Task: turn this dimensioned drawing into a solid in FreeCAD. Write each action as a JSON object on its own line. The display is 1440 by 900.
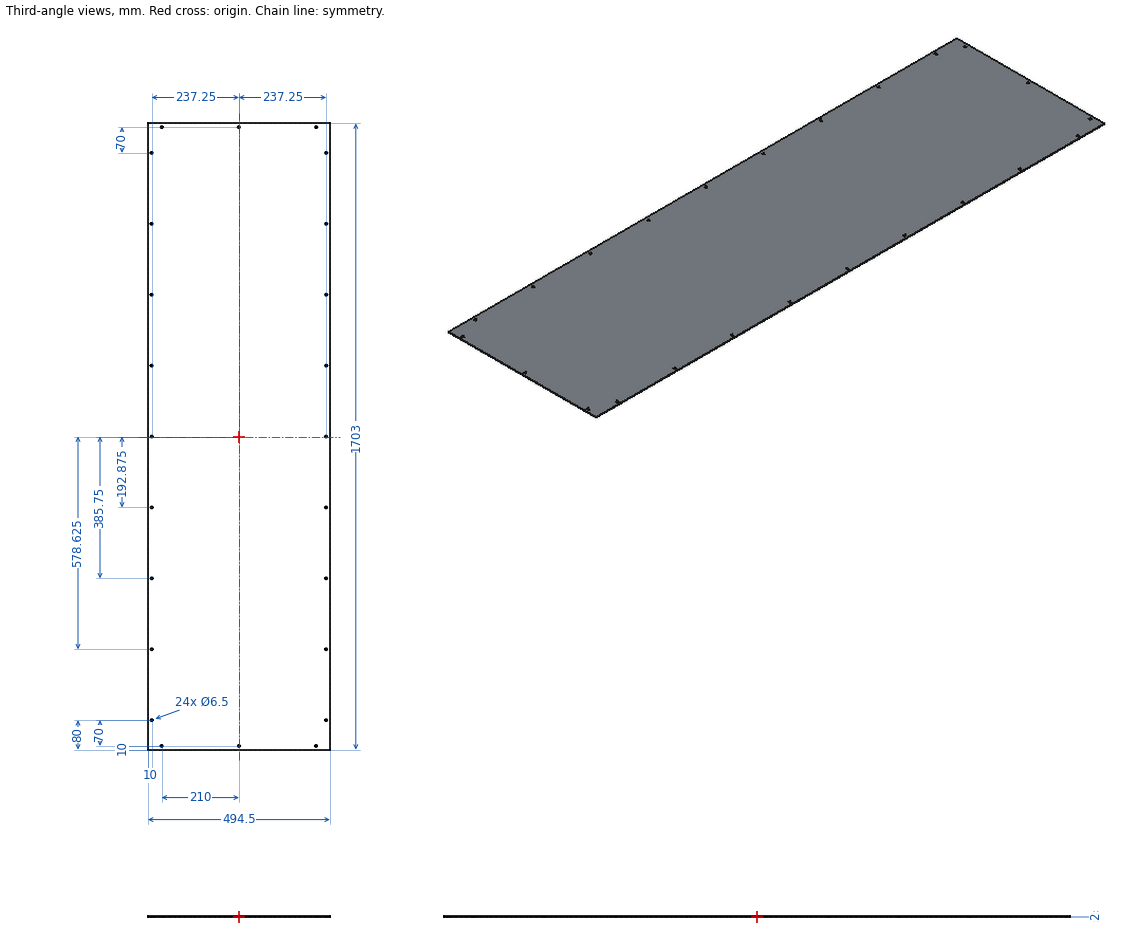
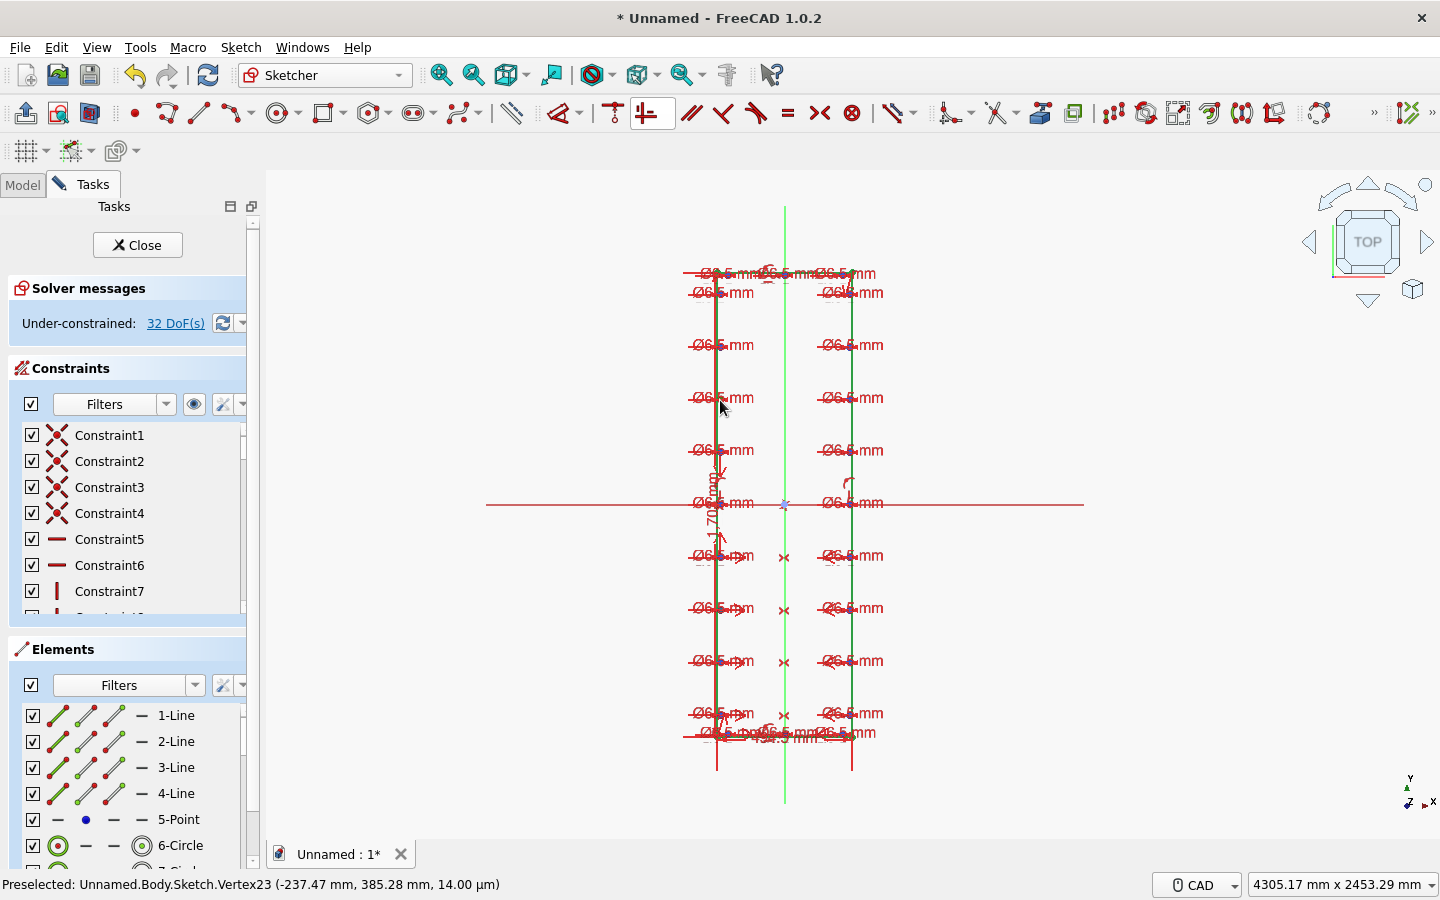
{"action": "left_click", "coordinate": [504, 505]}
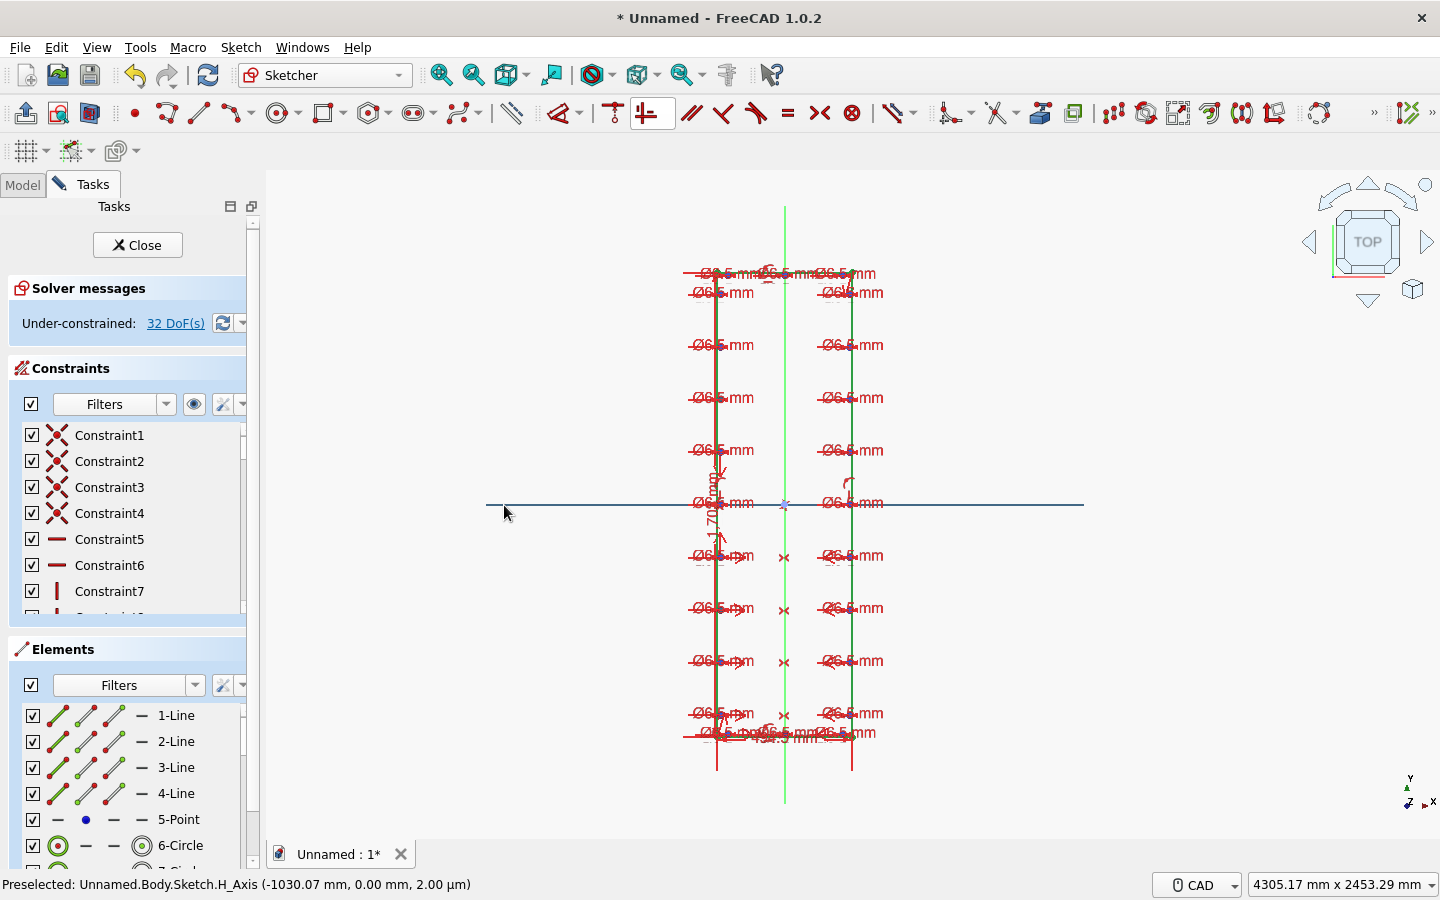
{"action": "left_click", "coordinate": [820, 114]}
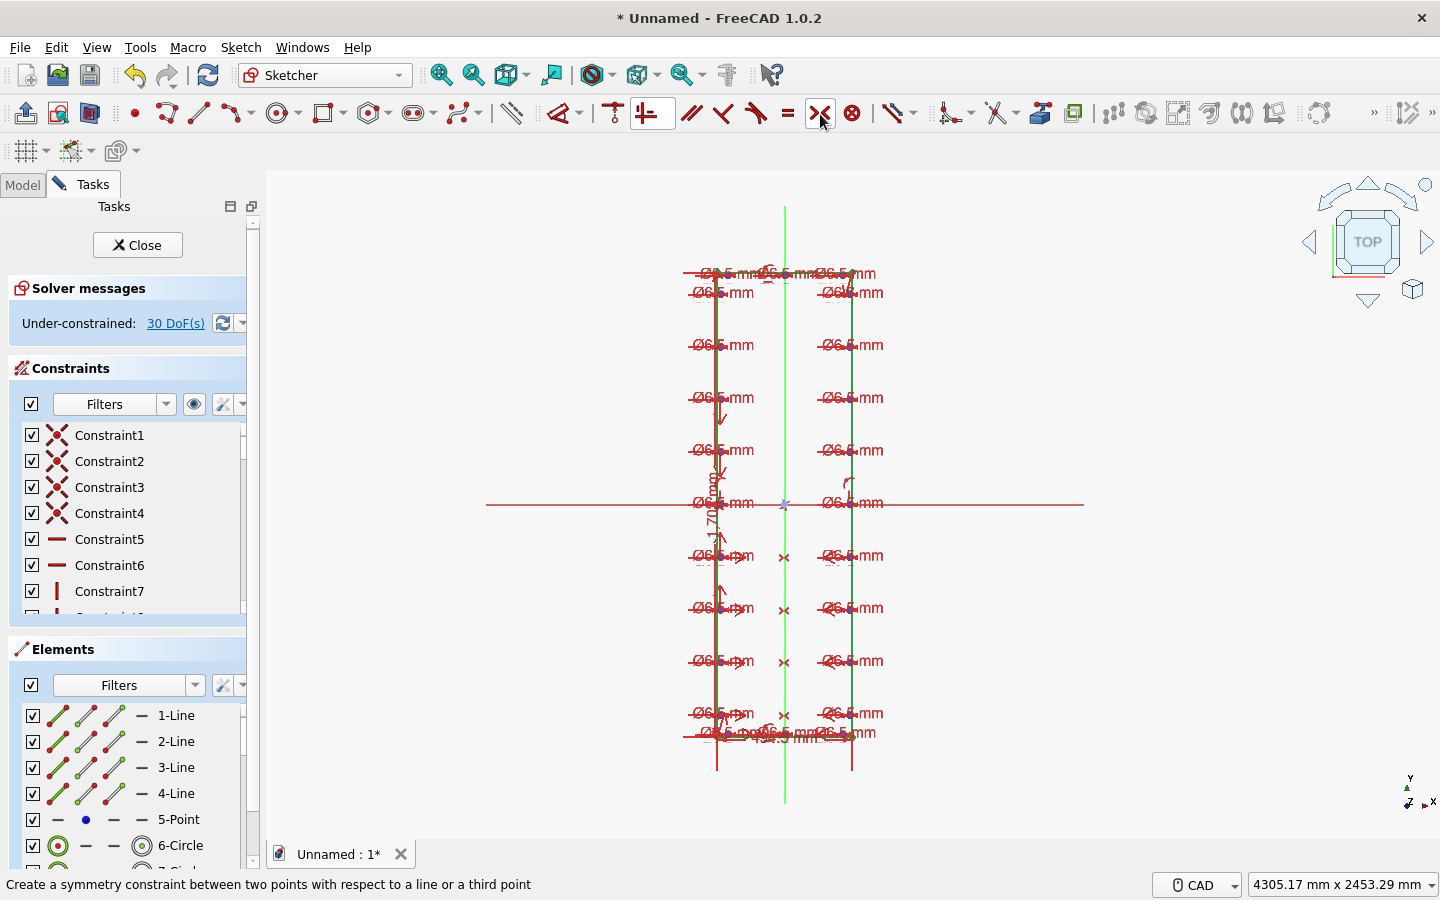
{"action": "left_click", "coordinate": [720, 663]}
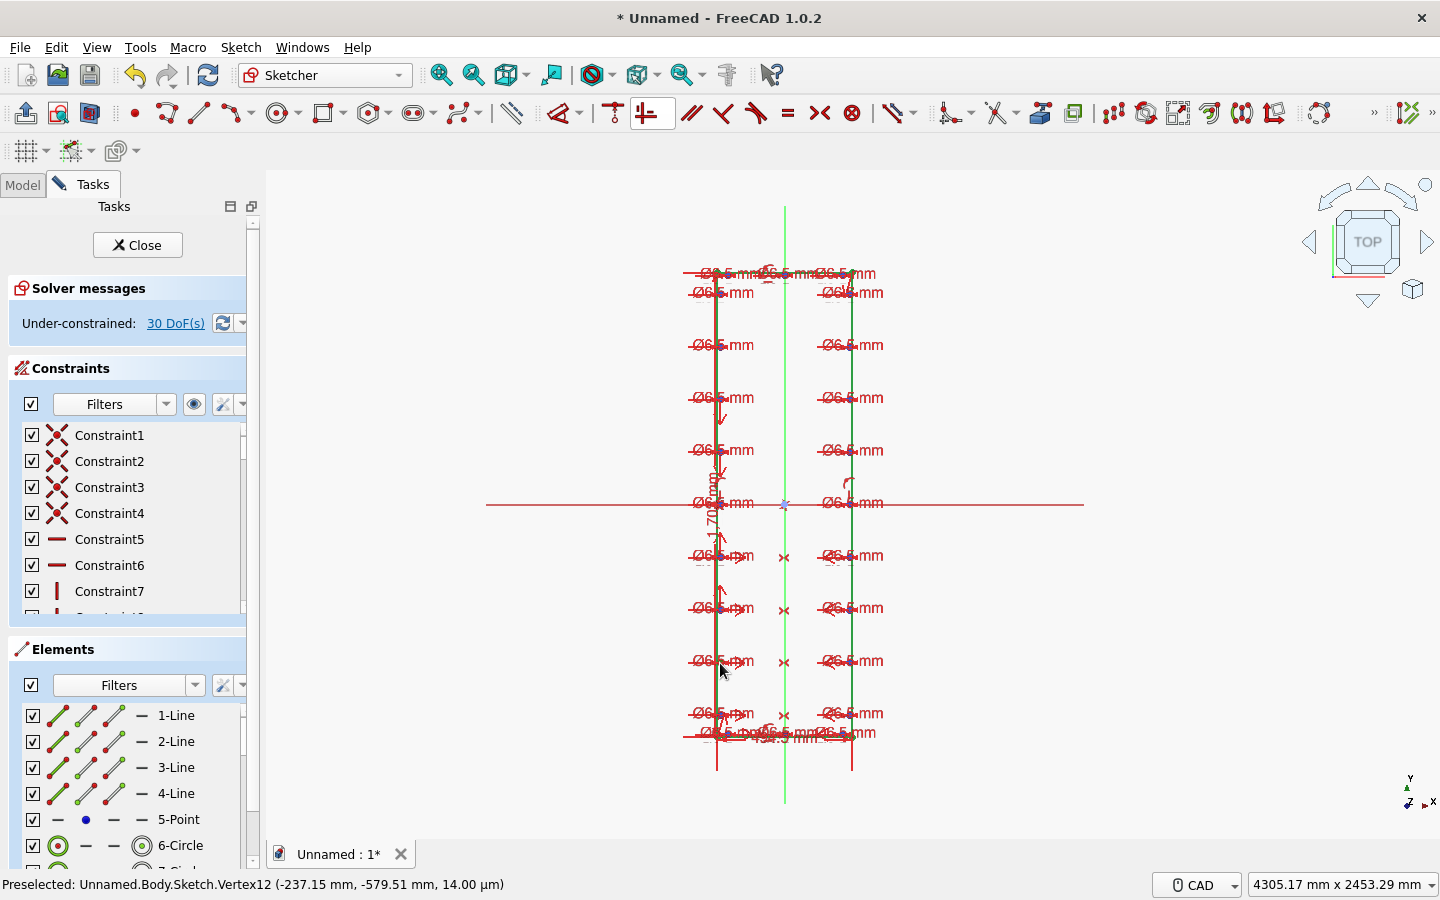
{"action": "left_click", "coordinate": [720, 347]}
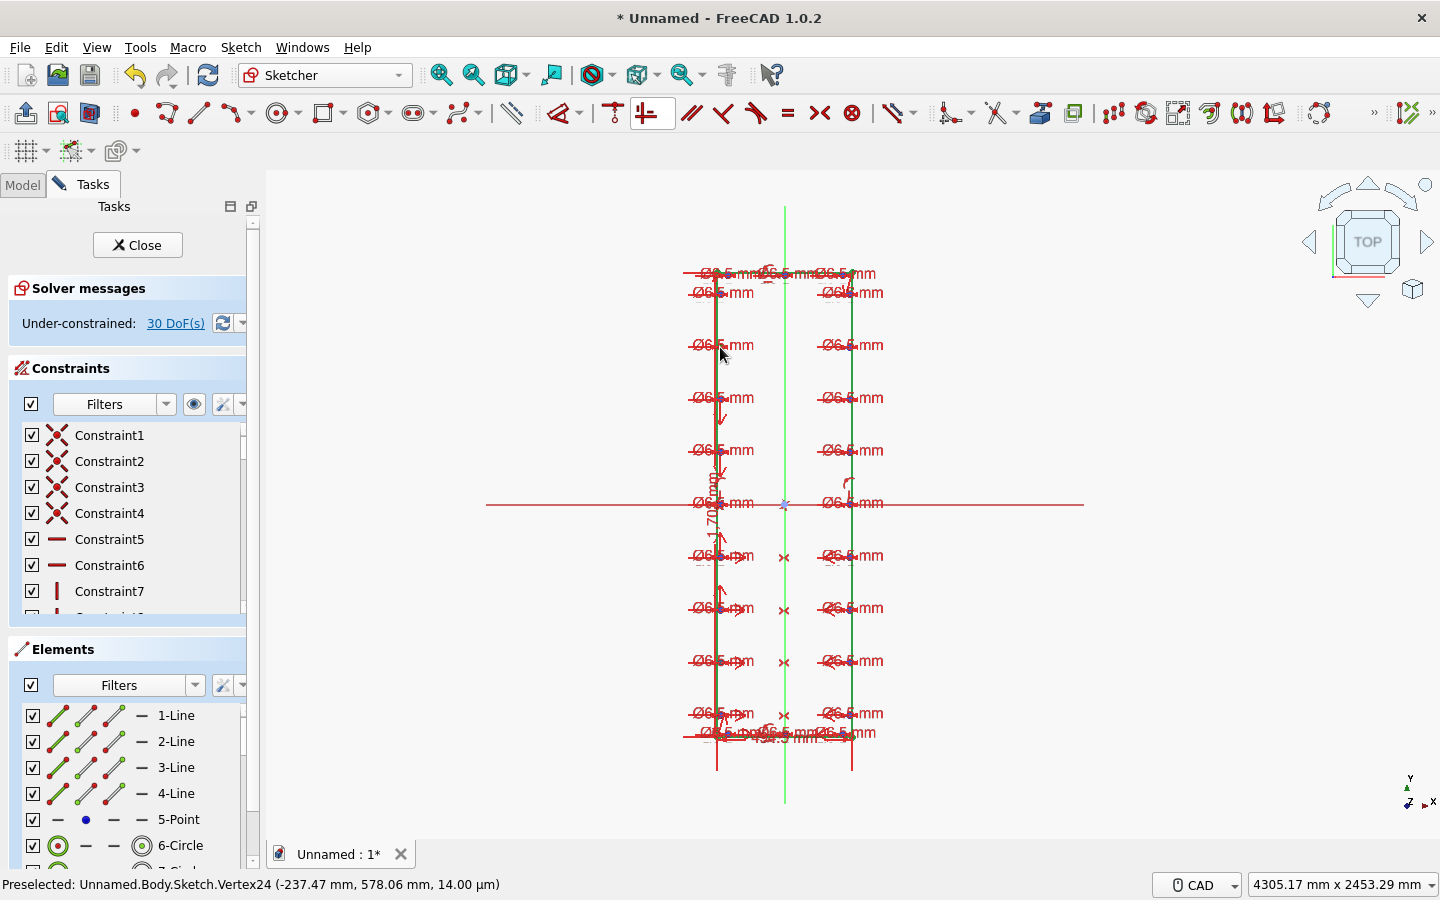
{"action": "left_click", "coordinate": [504, 505]}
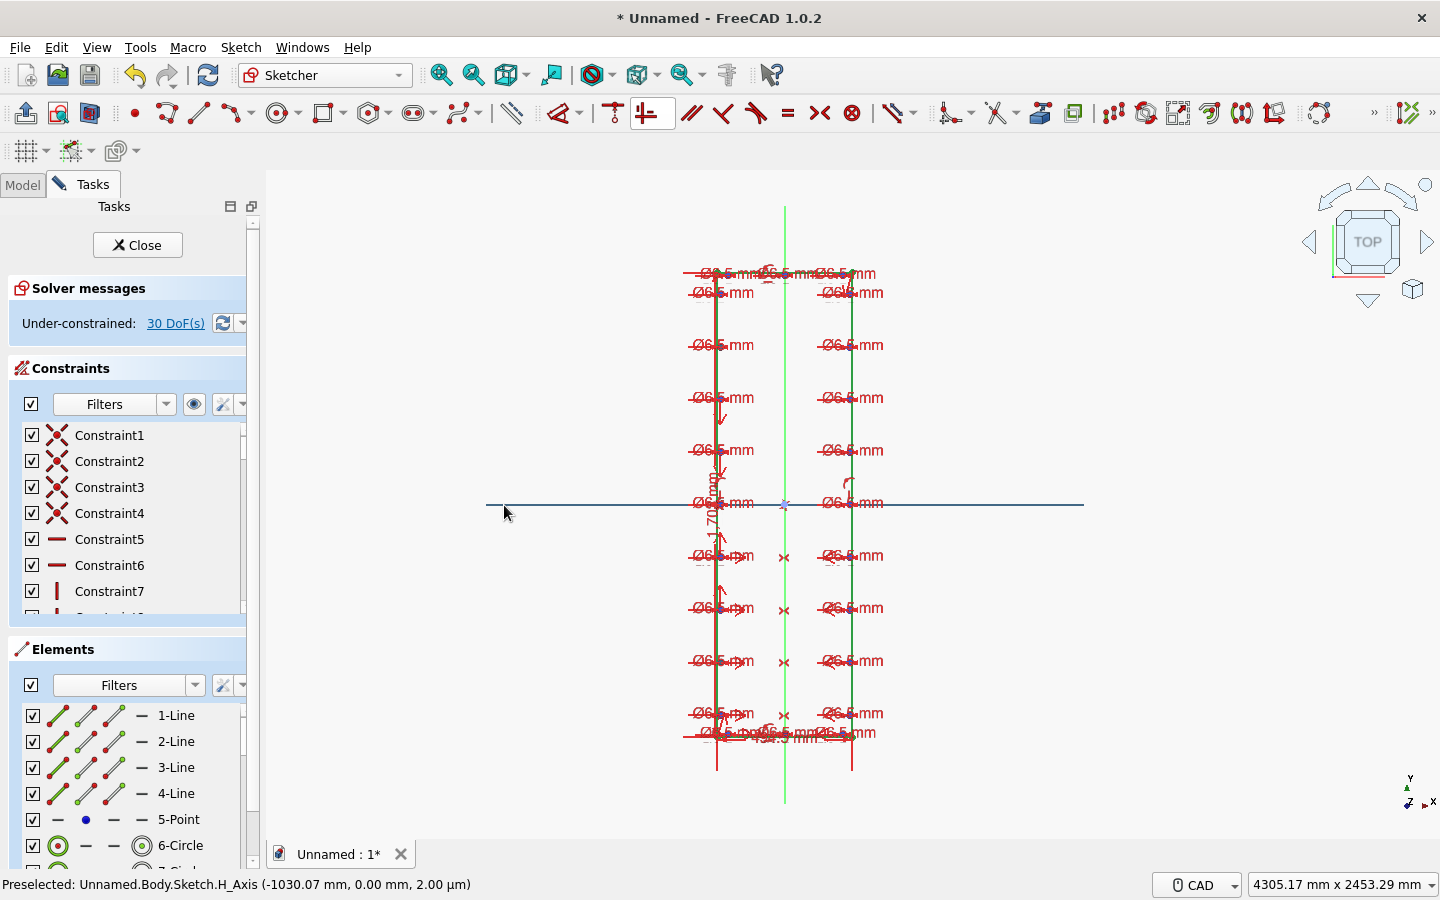
{"action": "left_click", "coordinate": [820, 114]}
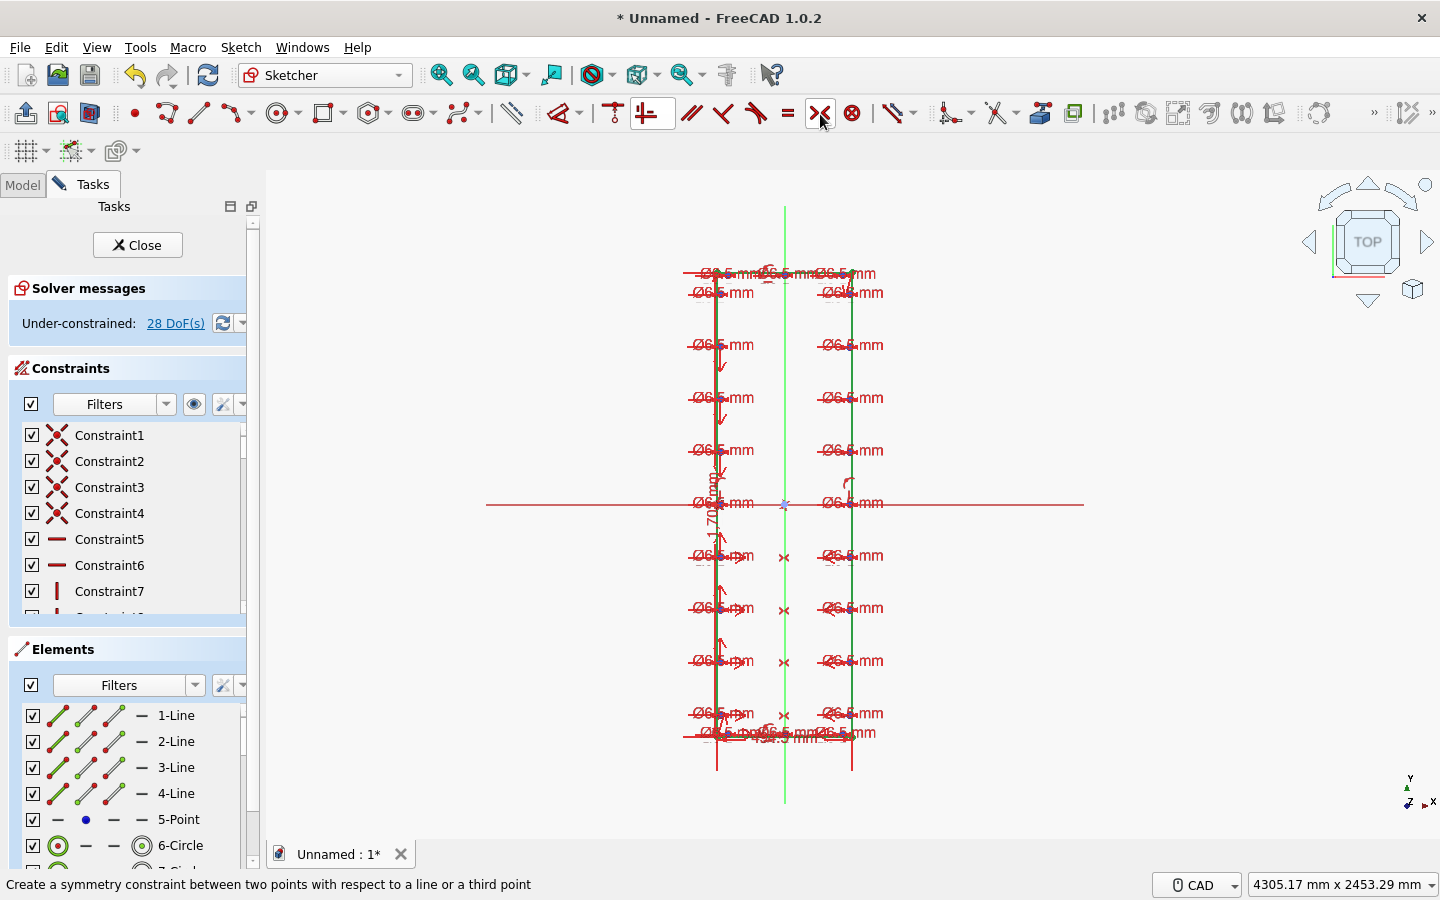
{"action": "left_click", "coordinate": [720, 715]}